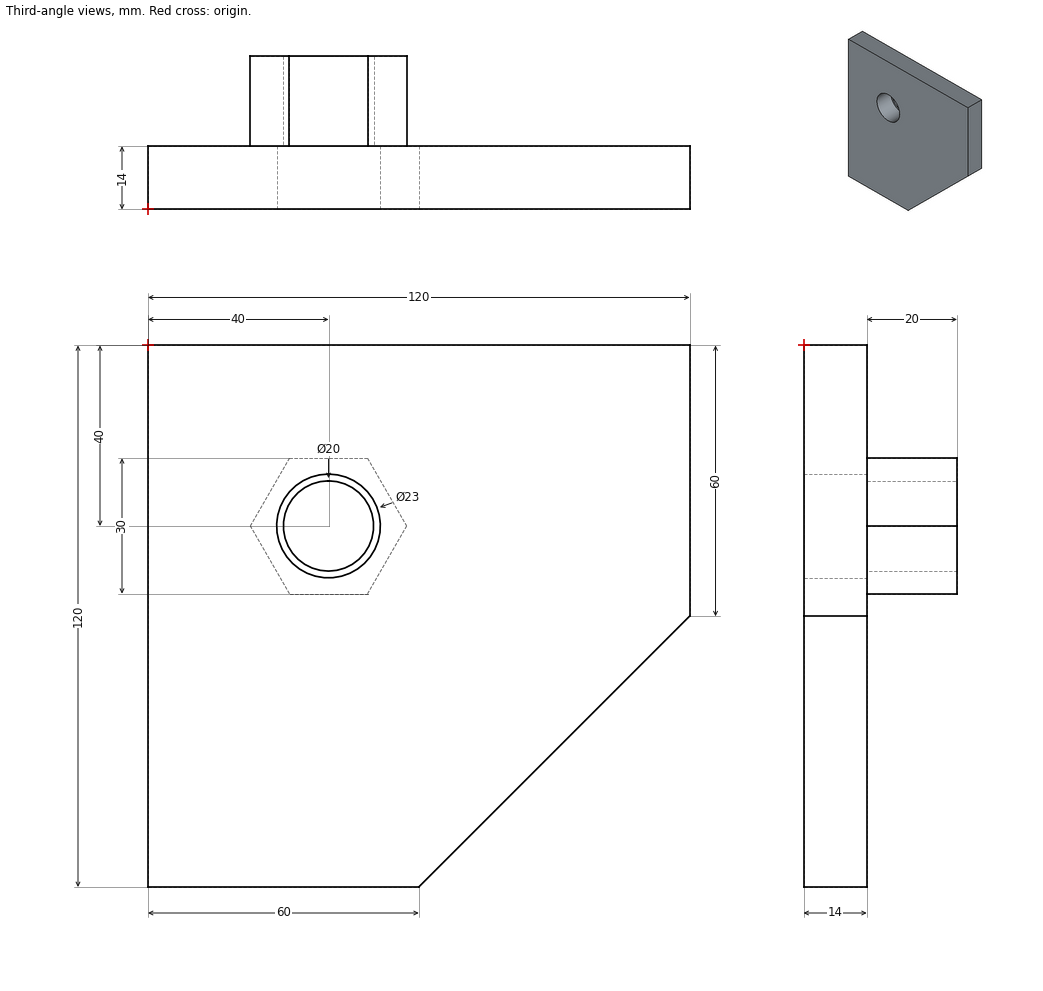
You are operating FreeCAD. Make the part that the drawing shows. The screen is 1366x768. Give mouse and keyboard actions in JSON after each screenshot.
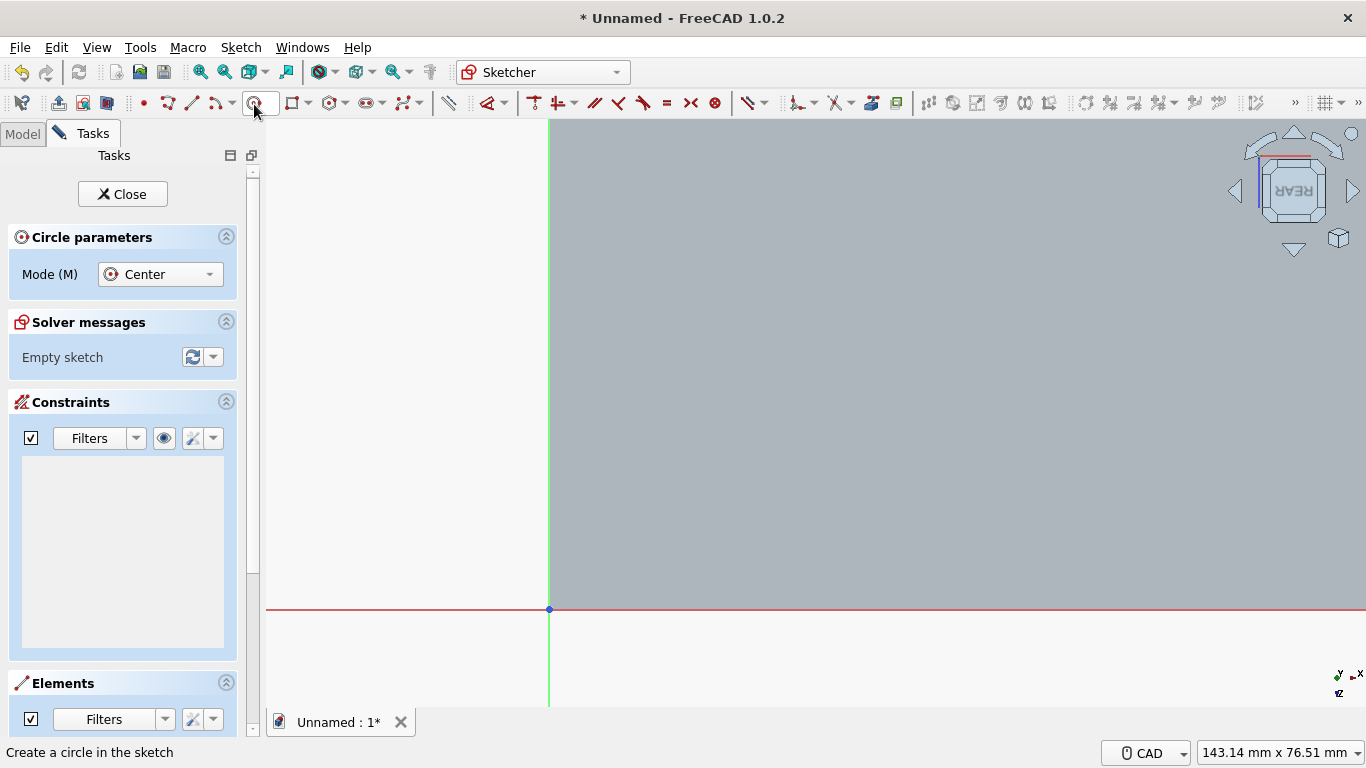
{"action": "left_click", "coordinate": [857, 302]}
{"action": "mouse_move", "coordinate": [919, 240]}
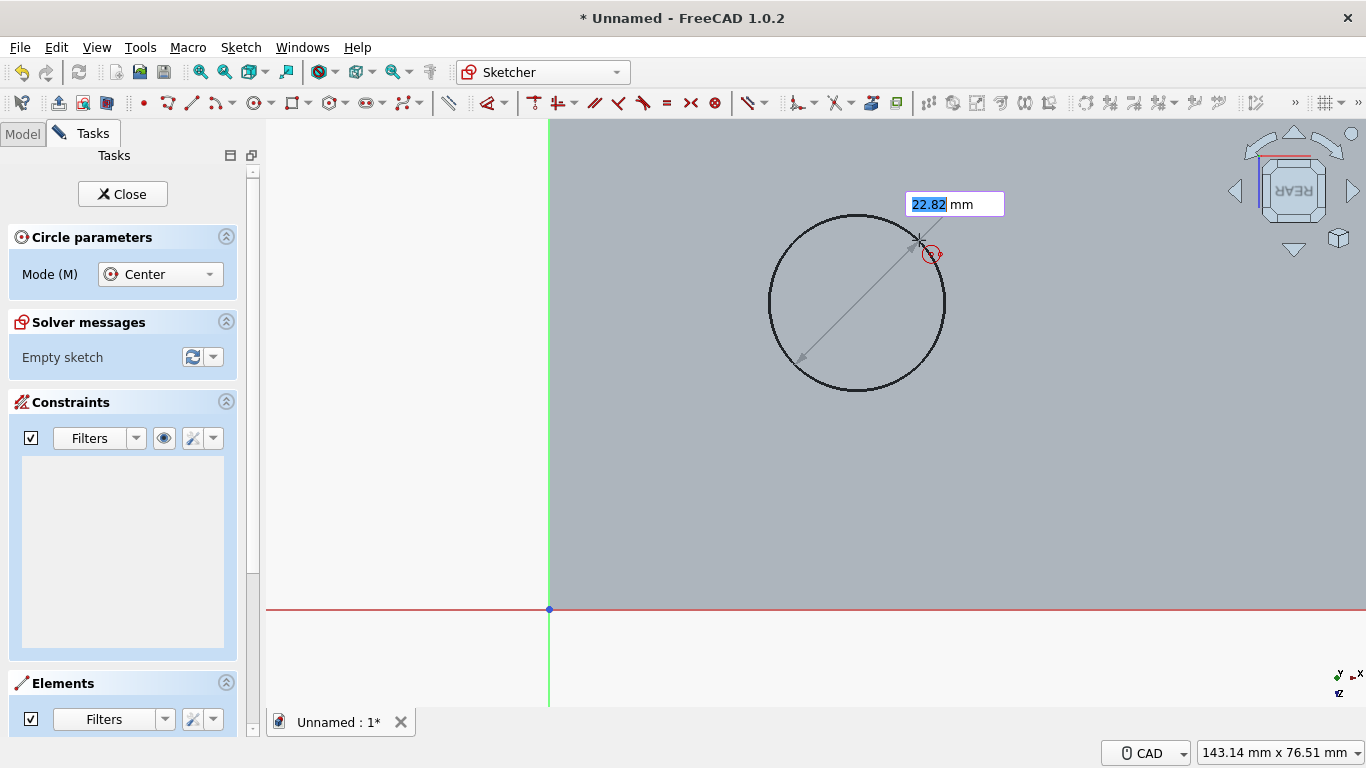
{"action": "type", "text": "23"}
{"action": "key", "text": "Return"}
{"action": "key", "text": "Escape"}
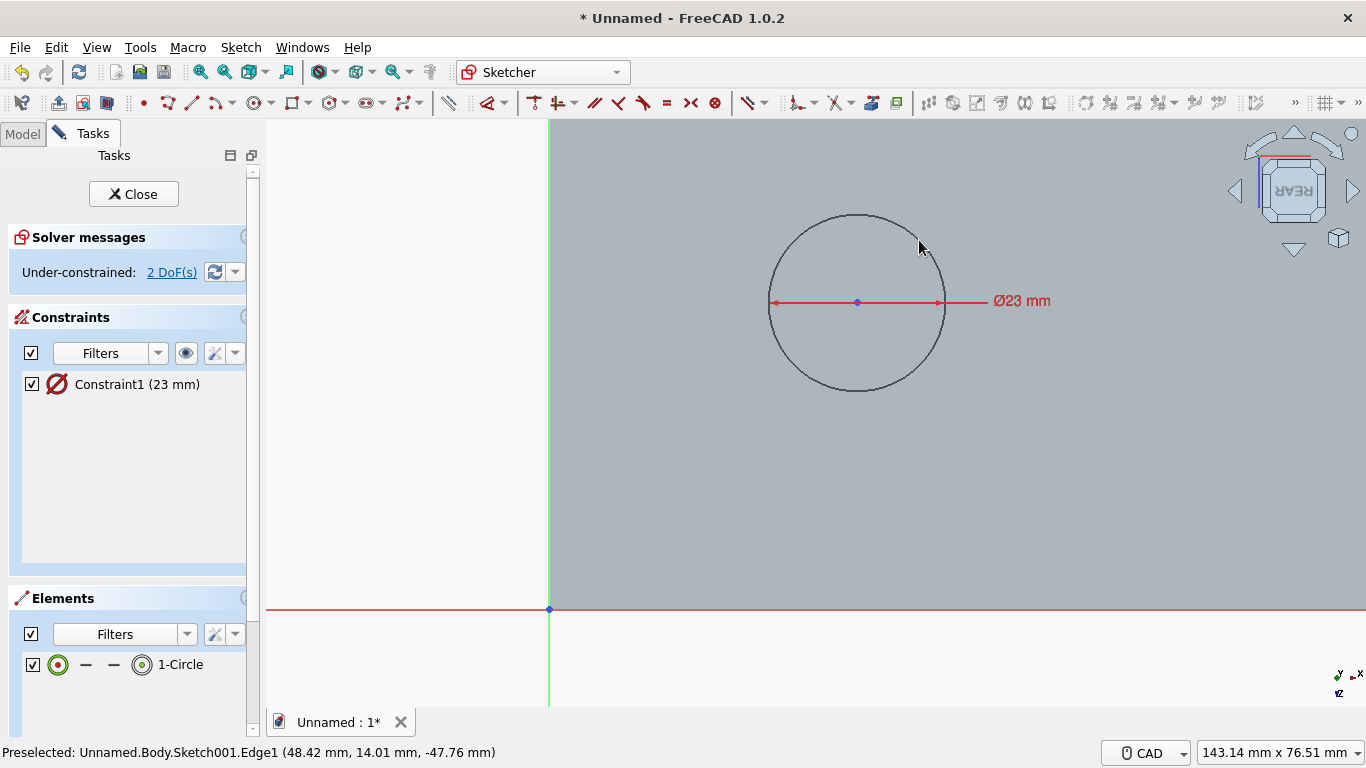
{"action": "left_click", "coordinate": [488, 104]}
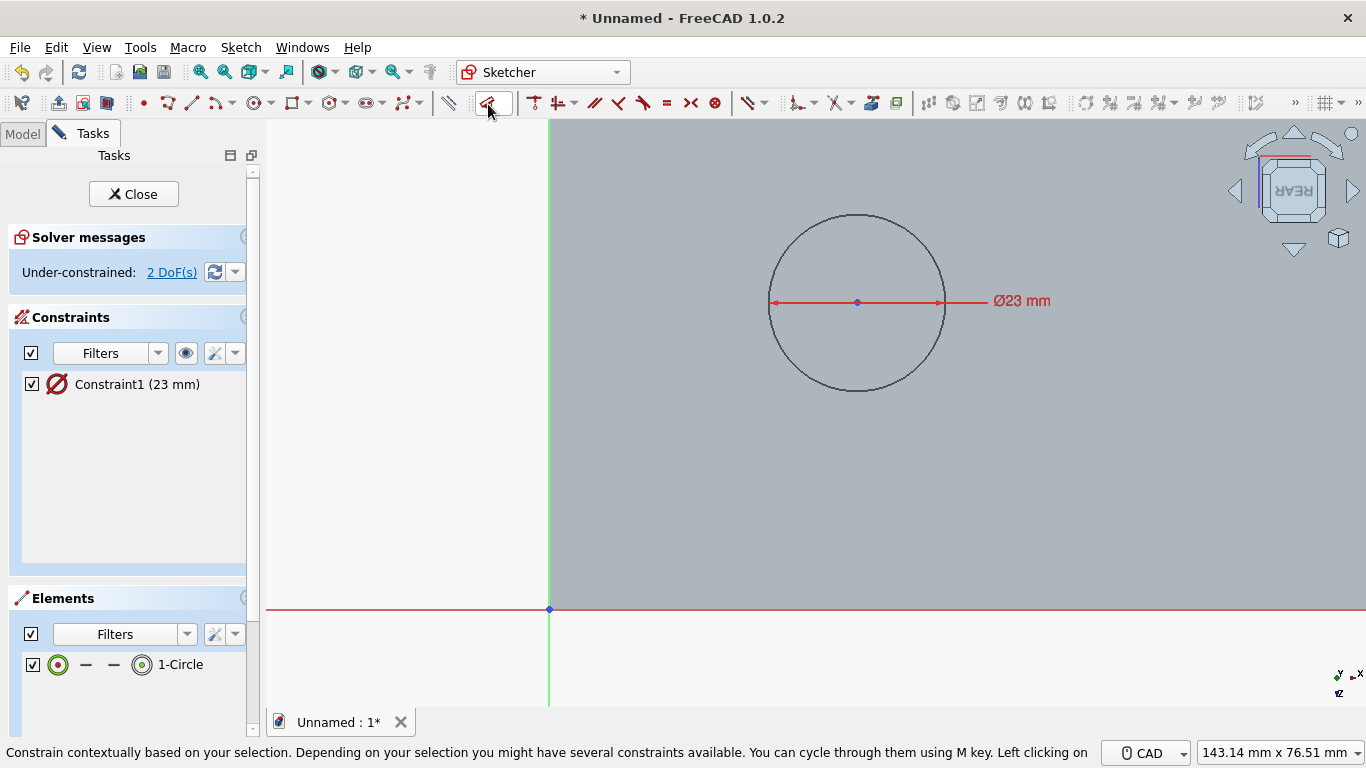
{"action": "left_click", "coordinate": [857, 303]}
{"action": "left_click", "coordinate": [703, 644]}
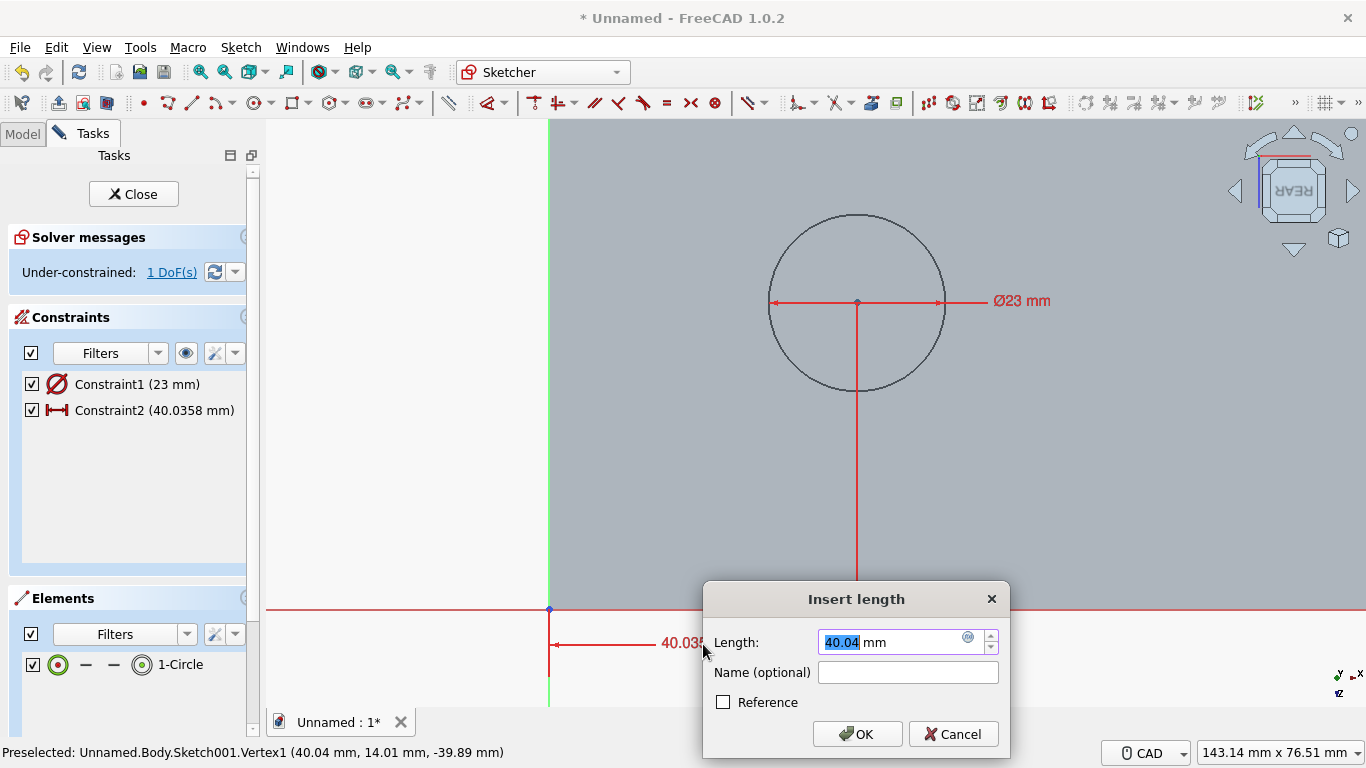
{"action": "type", "text": "40"}
{"action": "key", "text": "Return"}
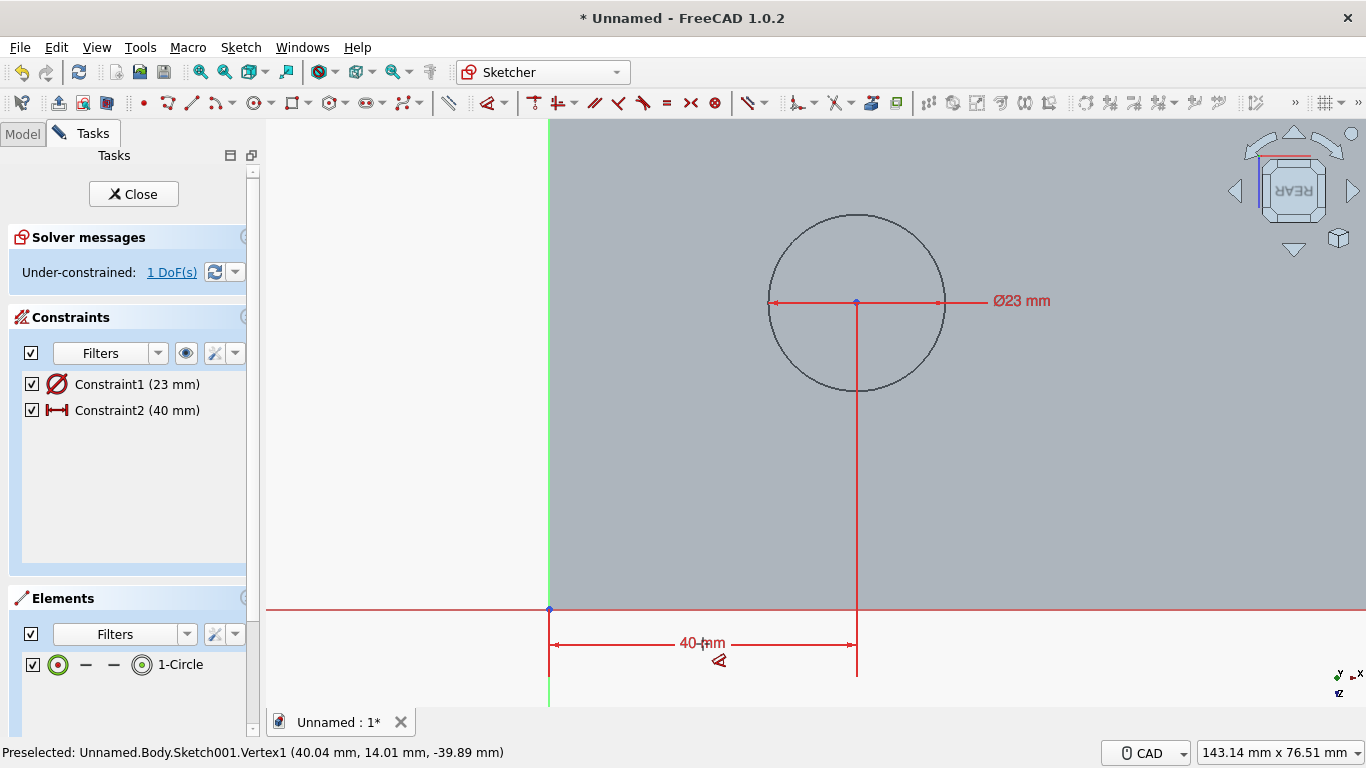
{"action": "left_click", "coordinate": [857, 303]}
{"action": "left_click", "coordinate": [515, 456]}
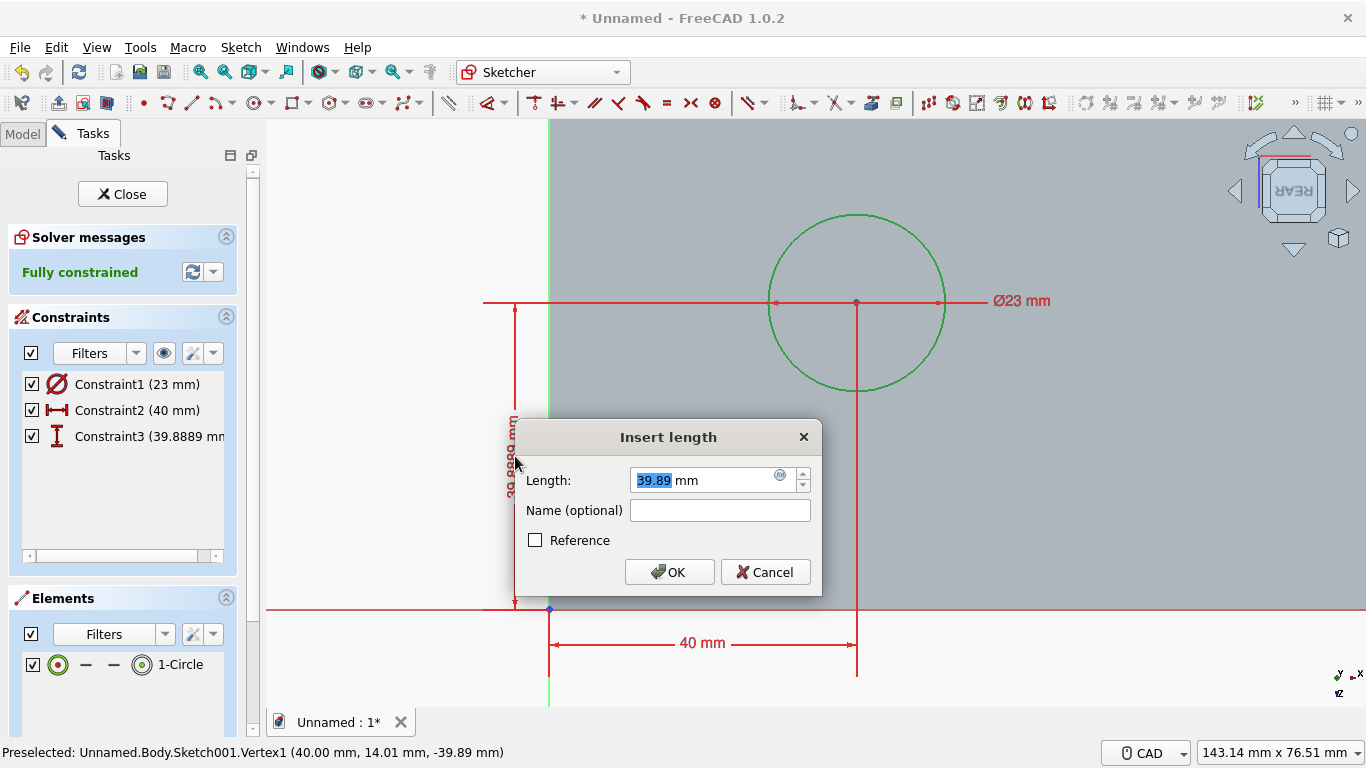
{"action": "type", "text": "40"}
{"action": "key", "text": "Return"}
{"action": "key", "text": "Escape"}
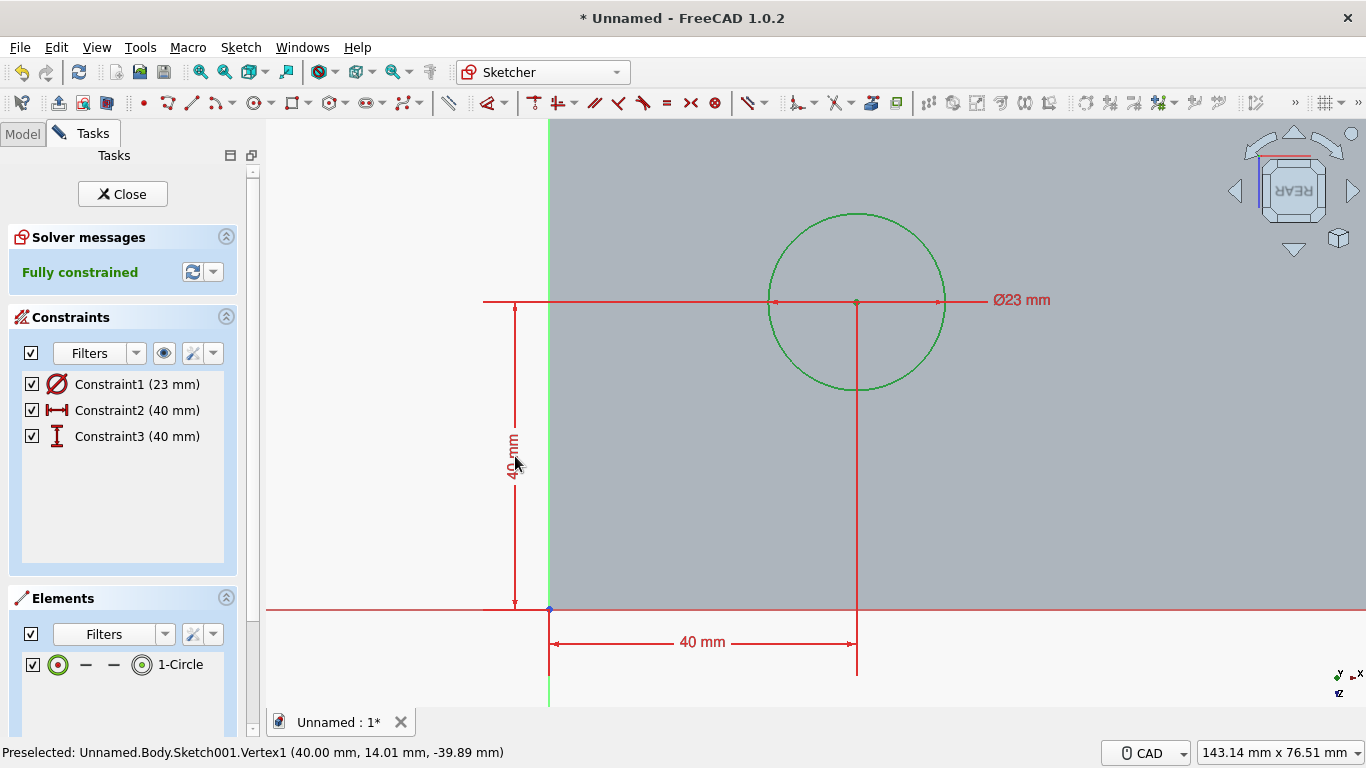
{"action": "left_click", "coordinate": [123, 194]}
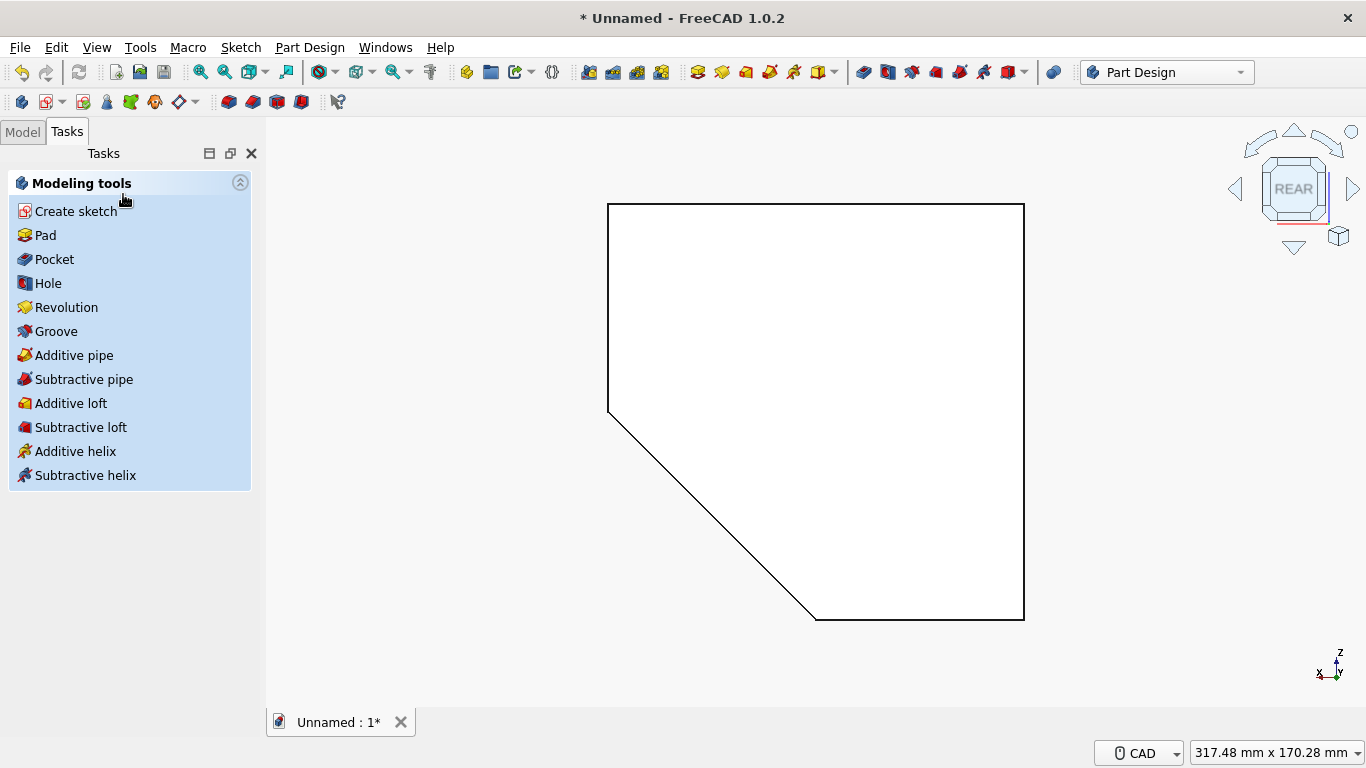
{"action": "left_click", "coordinate": [864, 72]}